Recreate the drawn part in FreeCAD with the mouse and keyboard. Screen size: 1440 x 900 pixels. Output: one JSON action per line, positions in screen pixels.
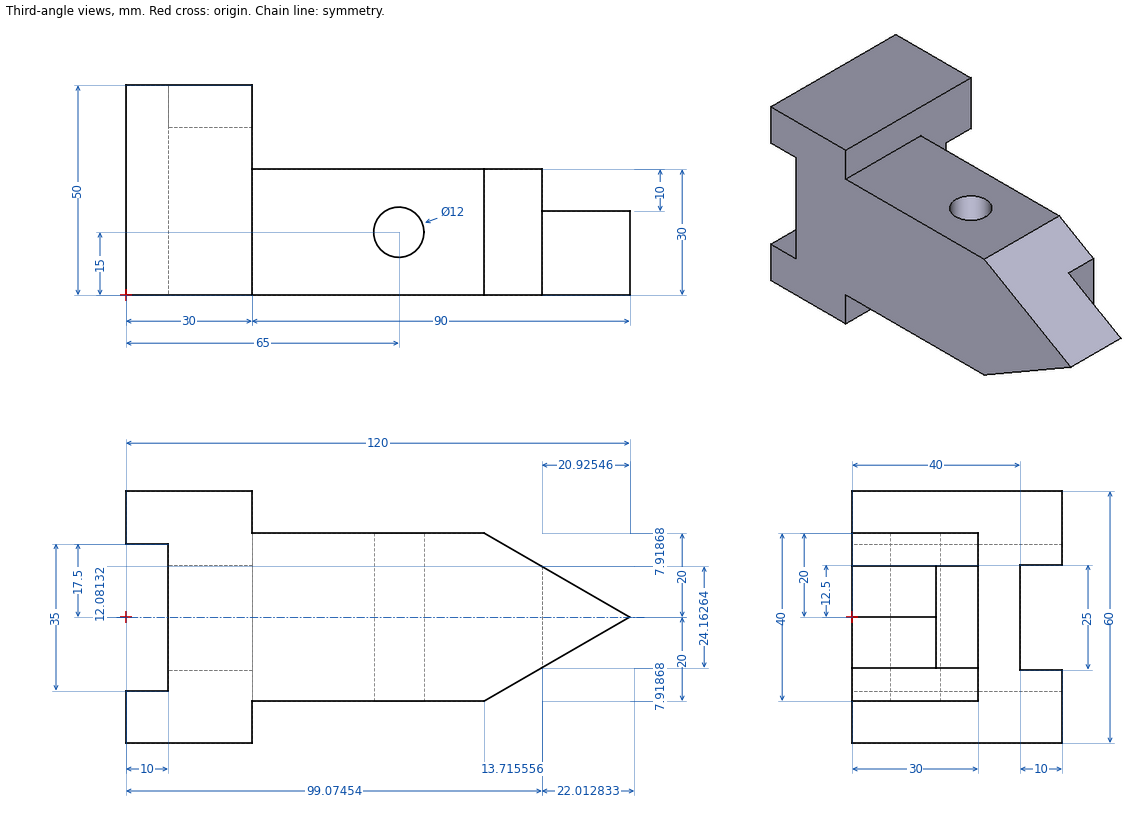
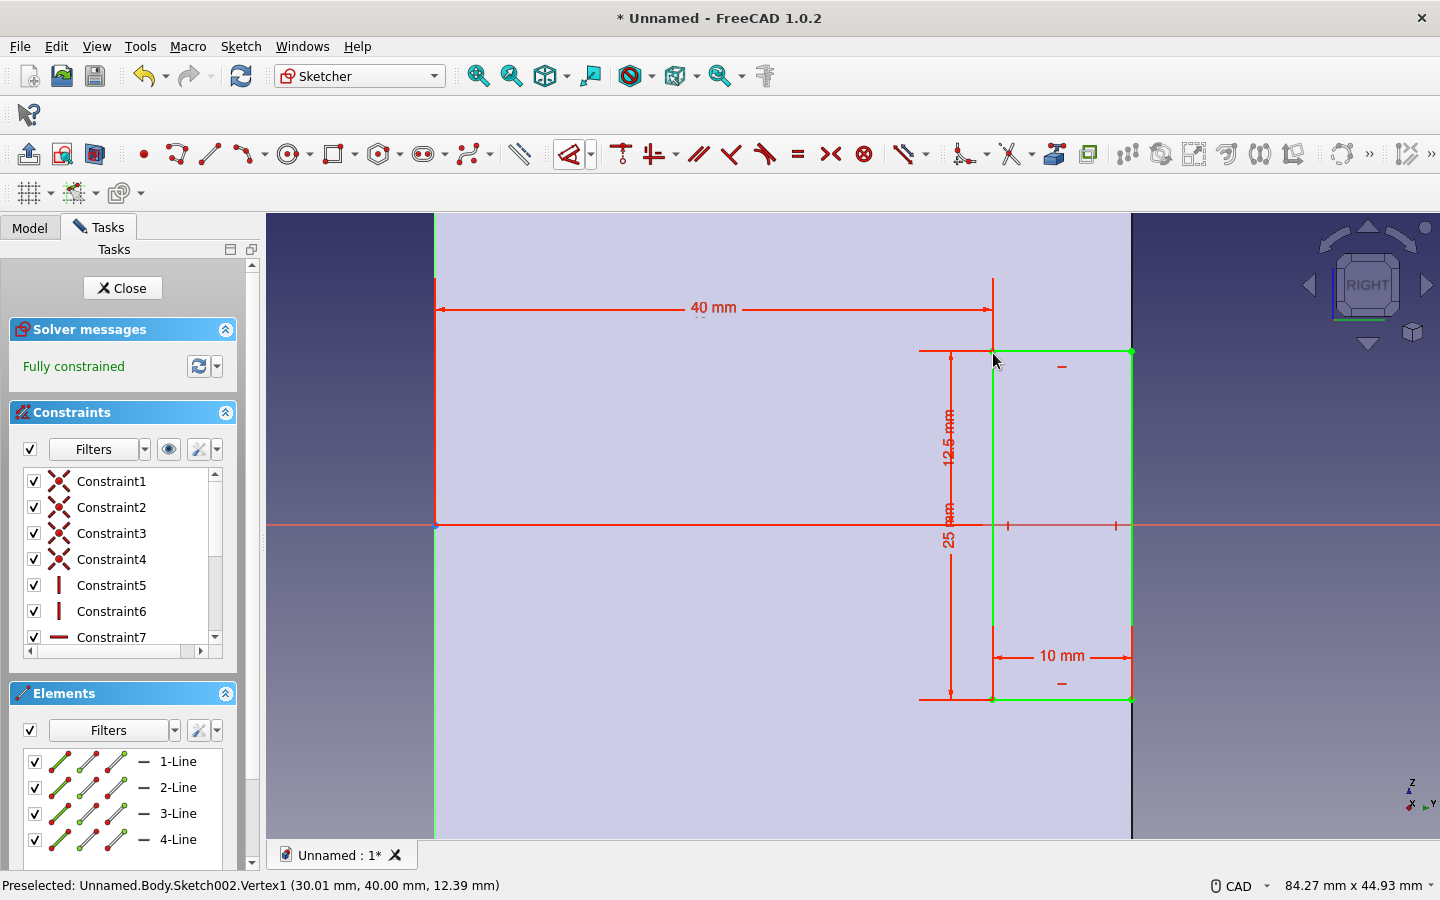
{"action": "left_click", "coordinate": [123, 288]}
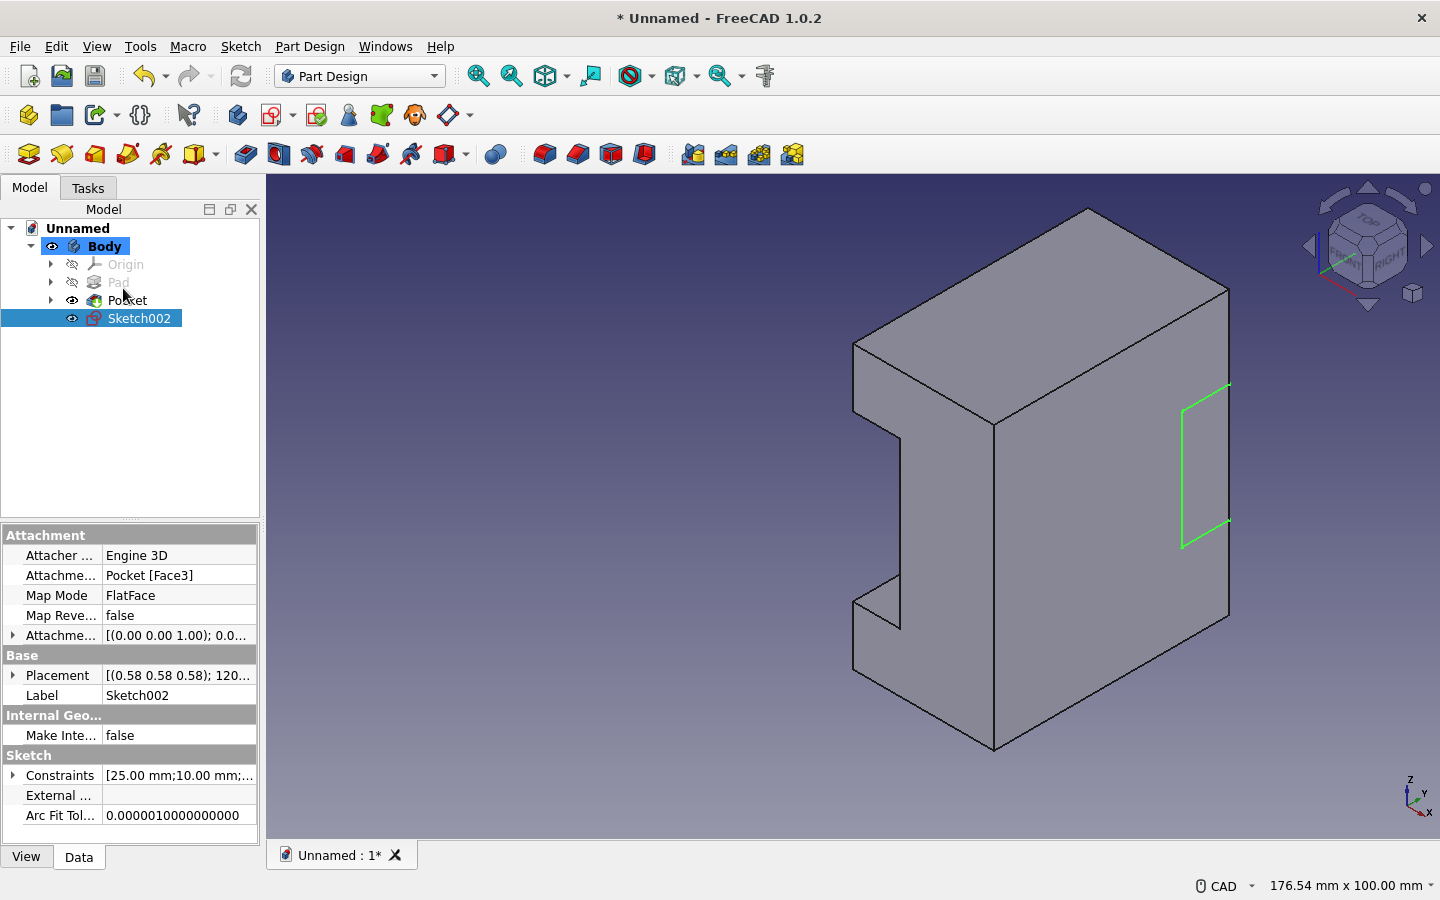
{"action": "left_click", "coordinate": [246, 154]}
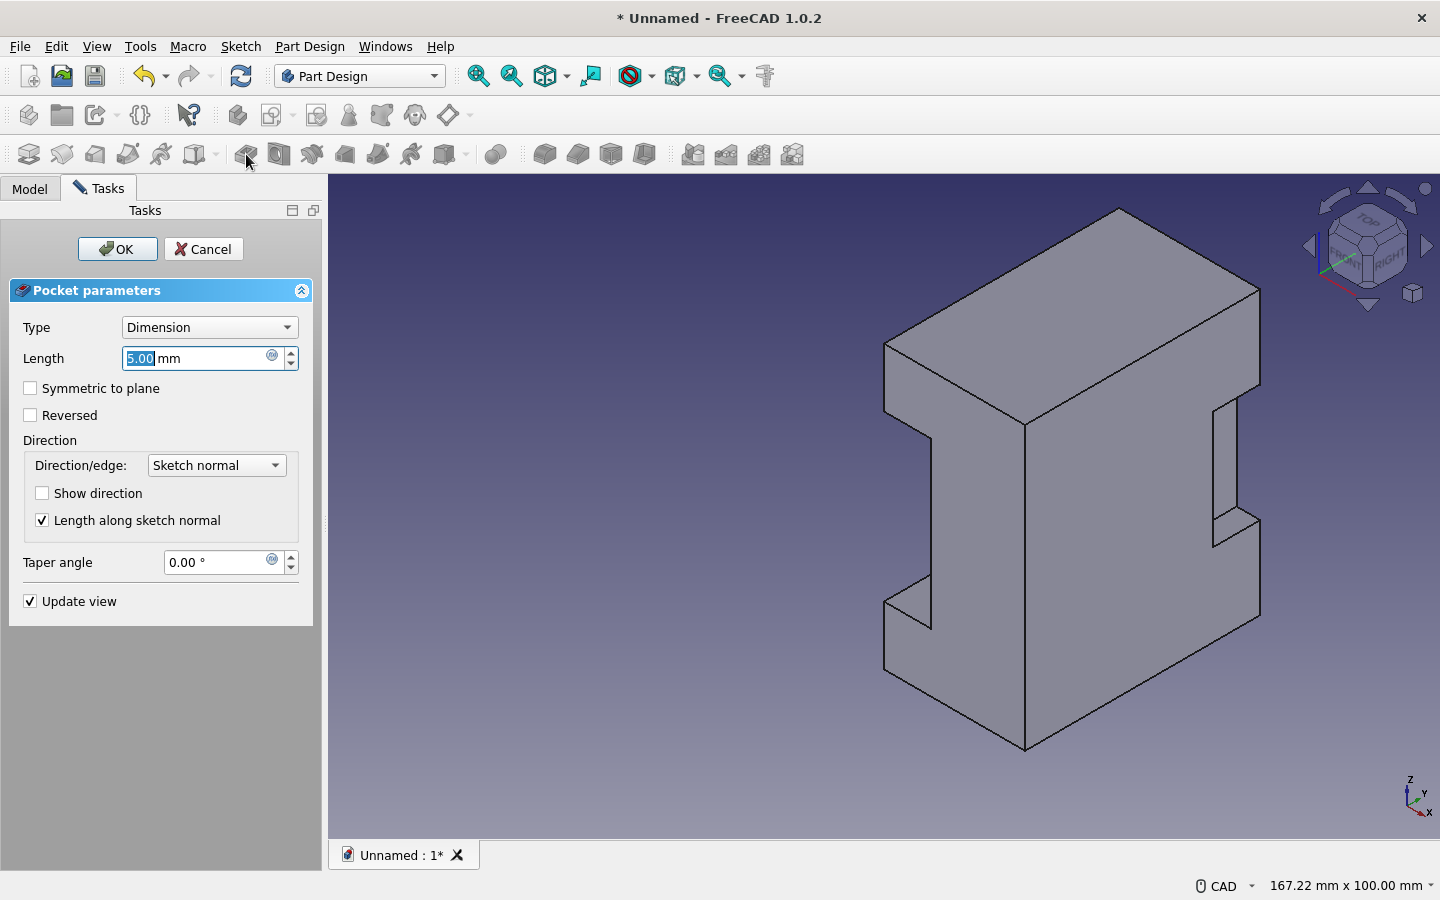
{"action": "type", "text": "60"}
{"action": "key", "text": "Tab"}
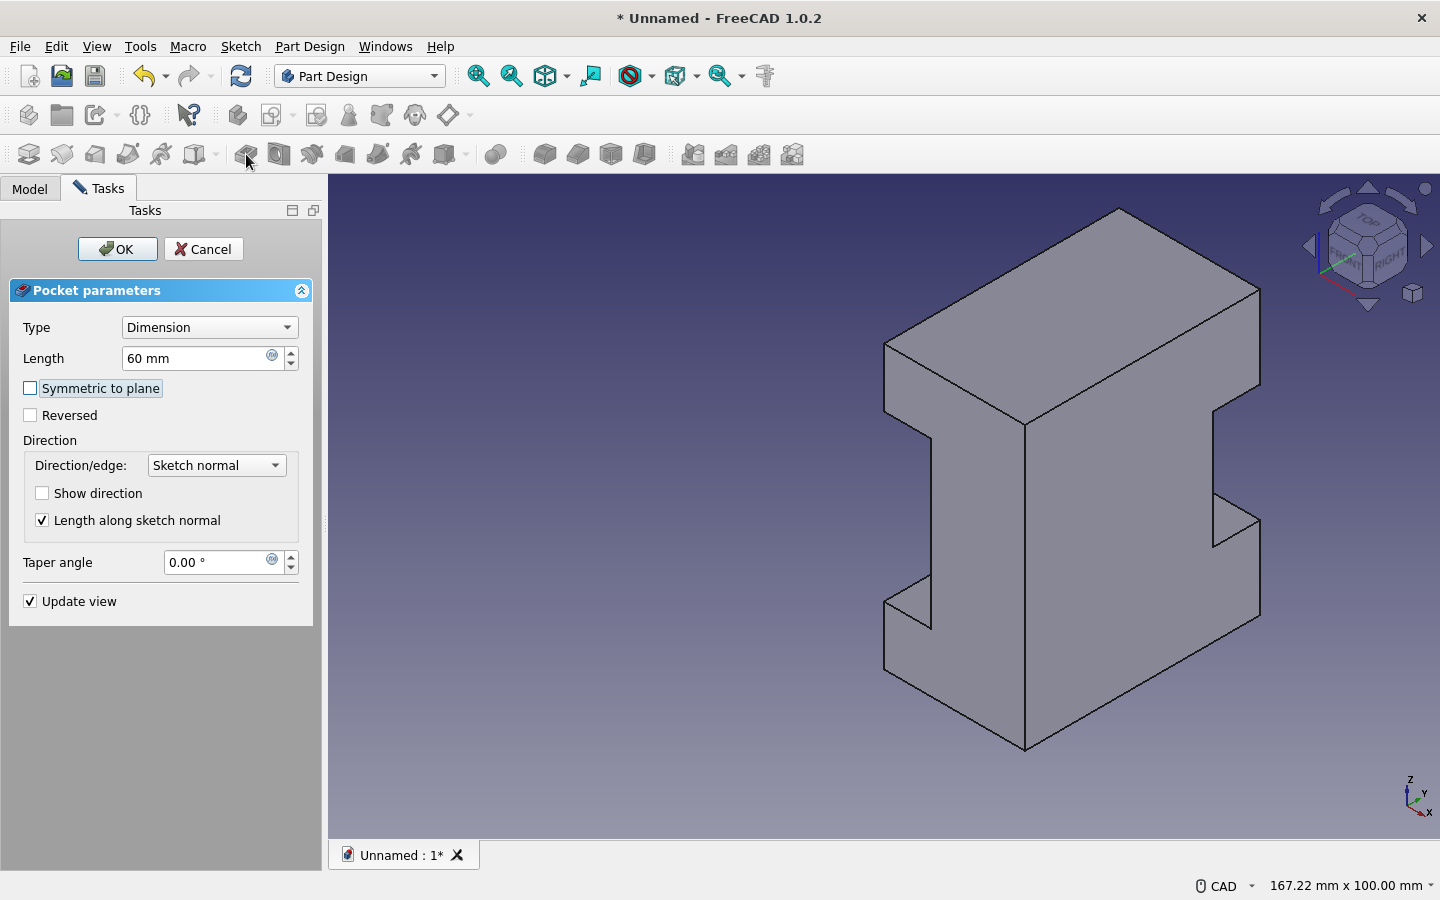
{"action": "left_click", "coordinate": [118, 249]}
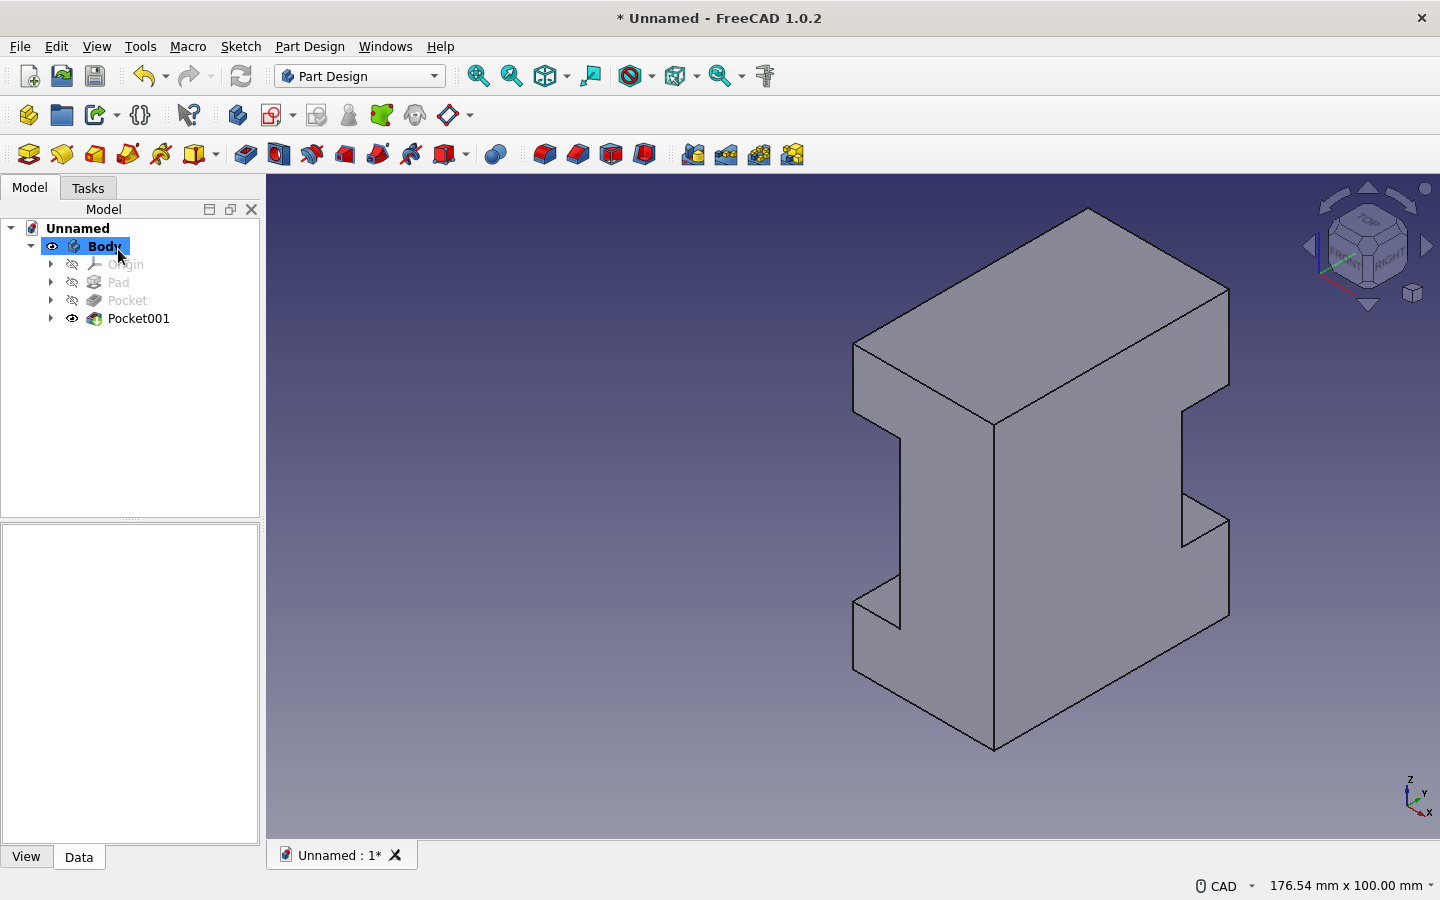
{"action": "left_click", "coordinate": [1078, 492]}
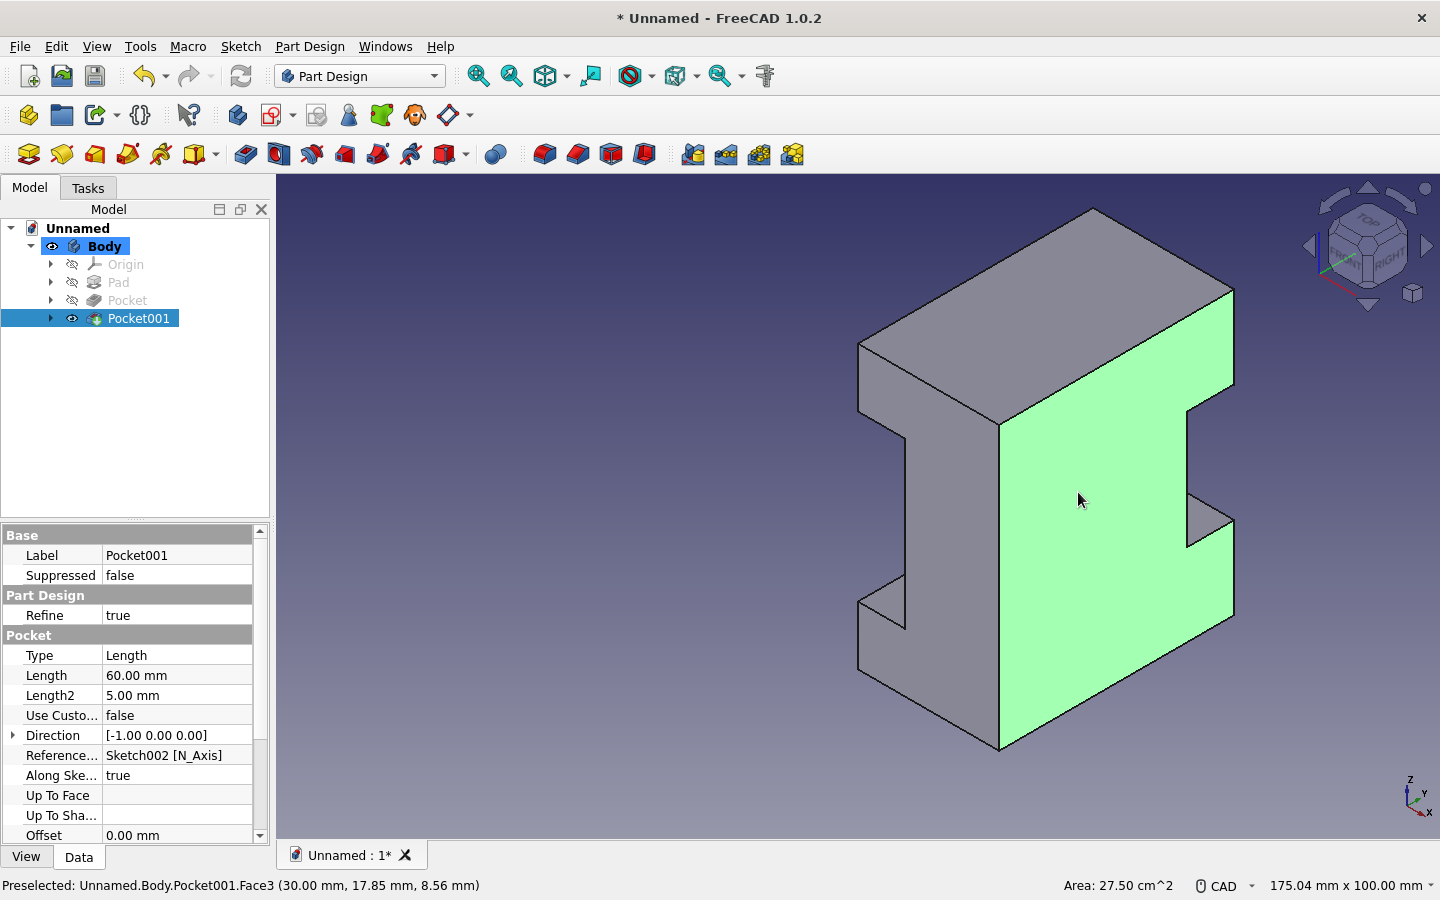
{"action": "left_click", "coordinate": [270, 116]}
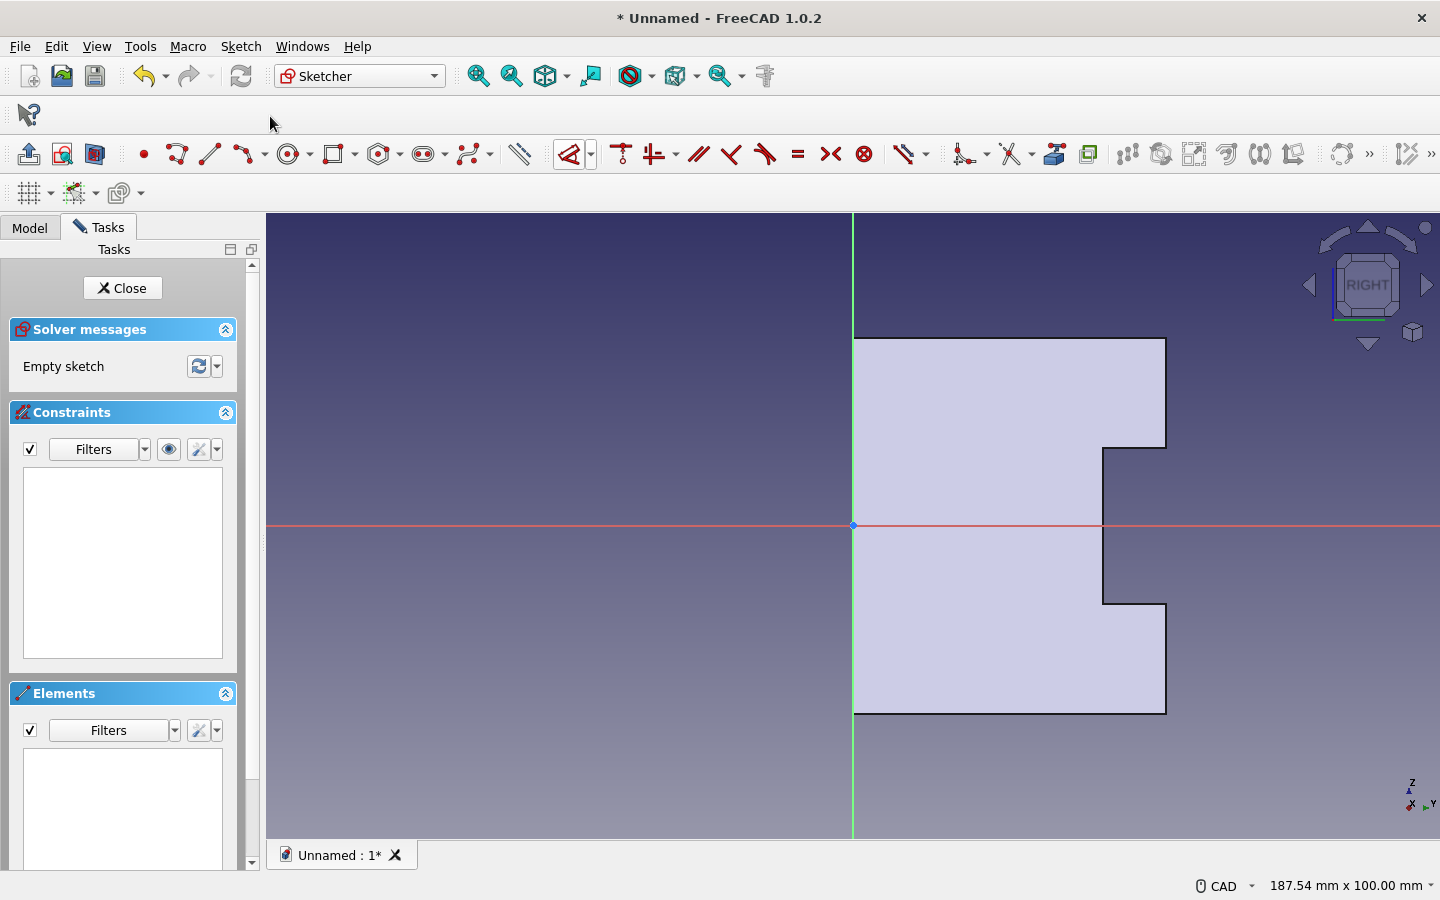
{"action": "scroll", "coordinate": [1275, 526], "scroll_direction": "up", "scroll_amount": 2}